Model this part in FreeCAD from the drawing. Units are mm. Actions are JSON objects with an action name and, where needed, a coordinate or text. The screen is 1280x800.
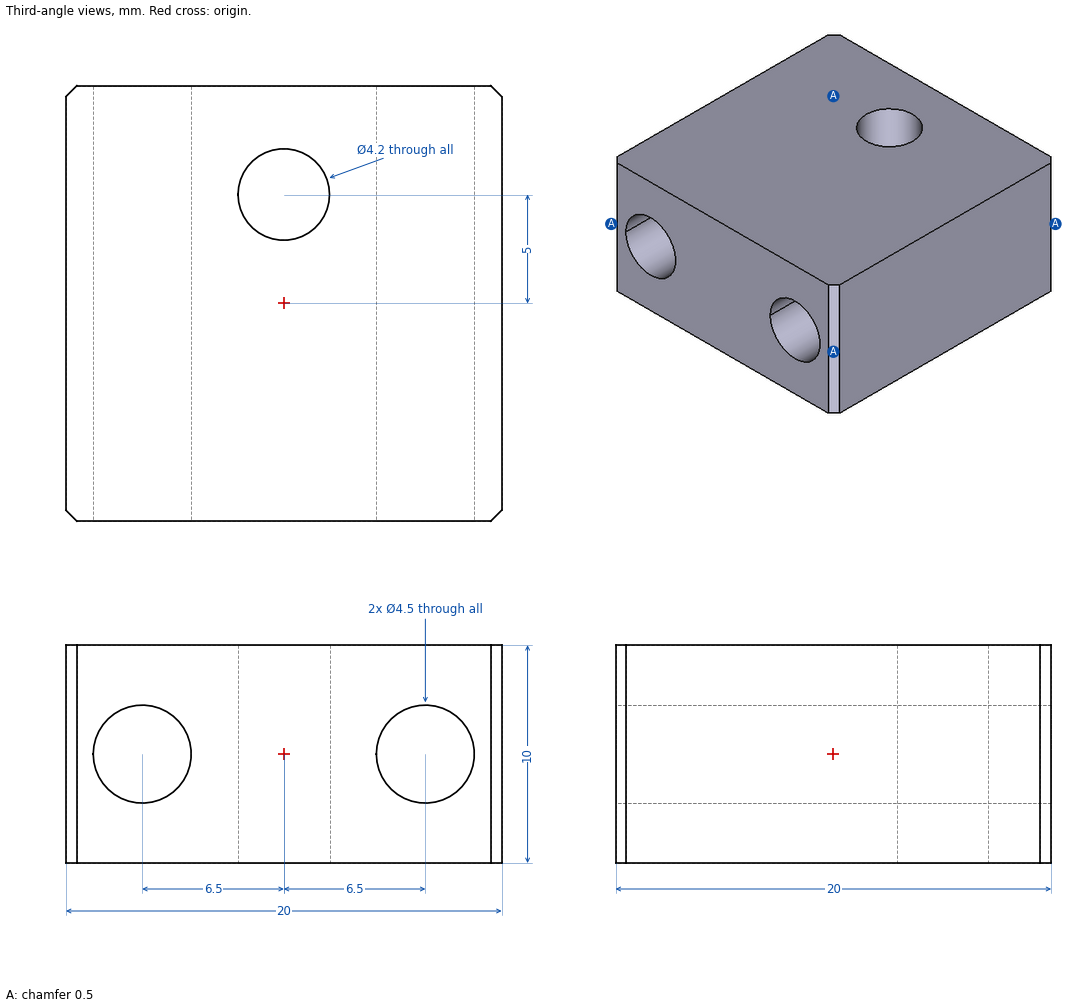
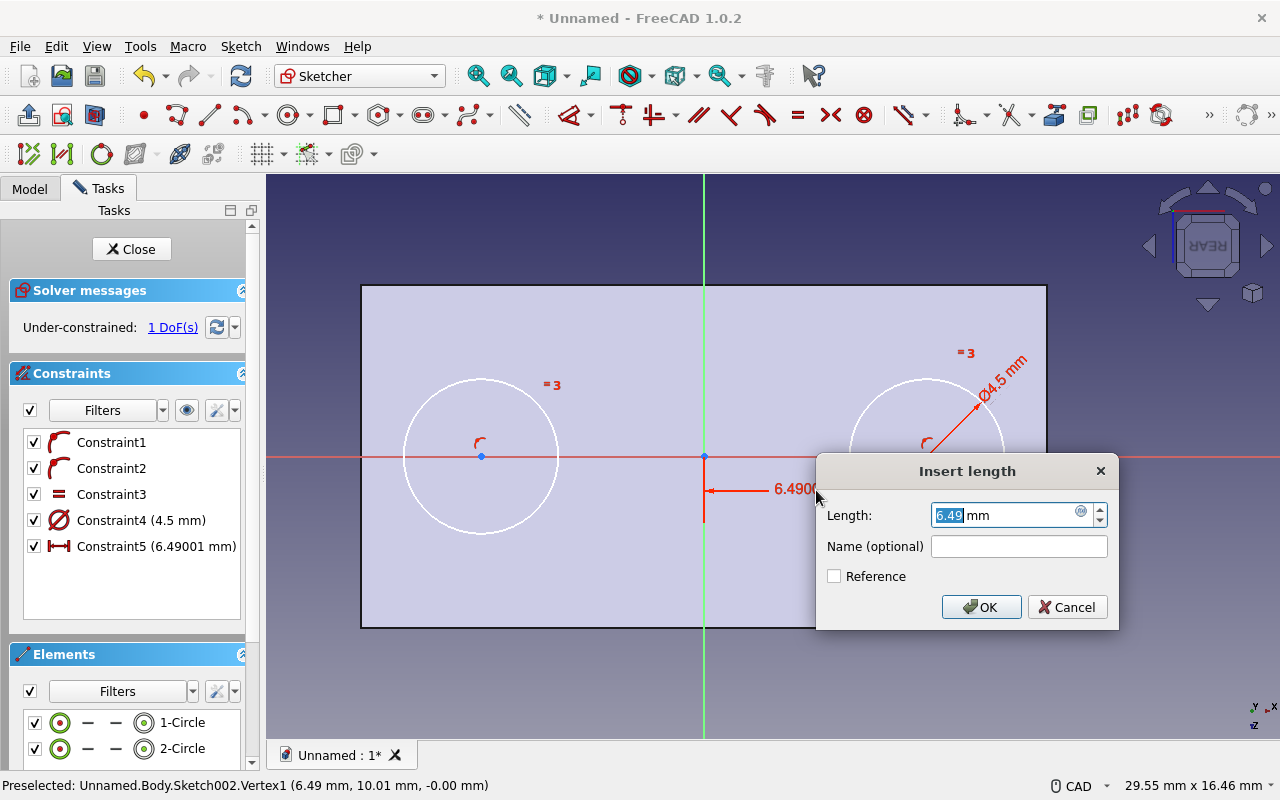
{"action": "type", "text": "6.5"}
{"action": "key", "text": "Return"}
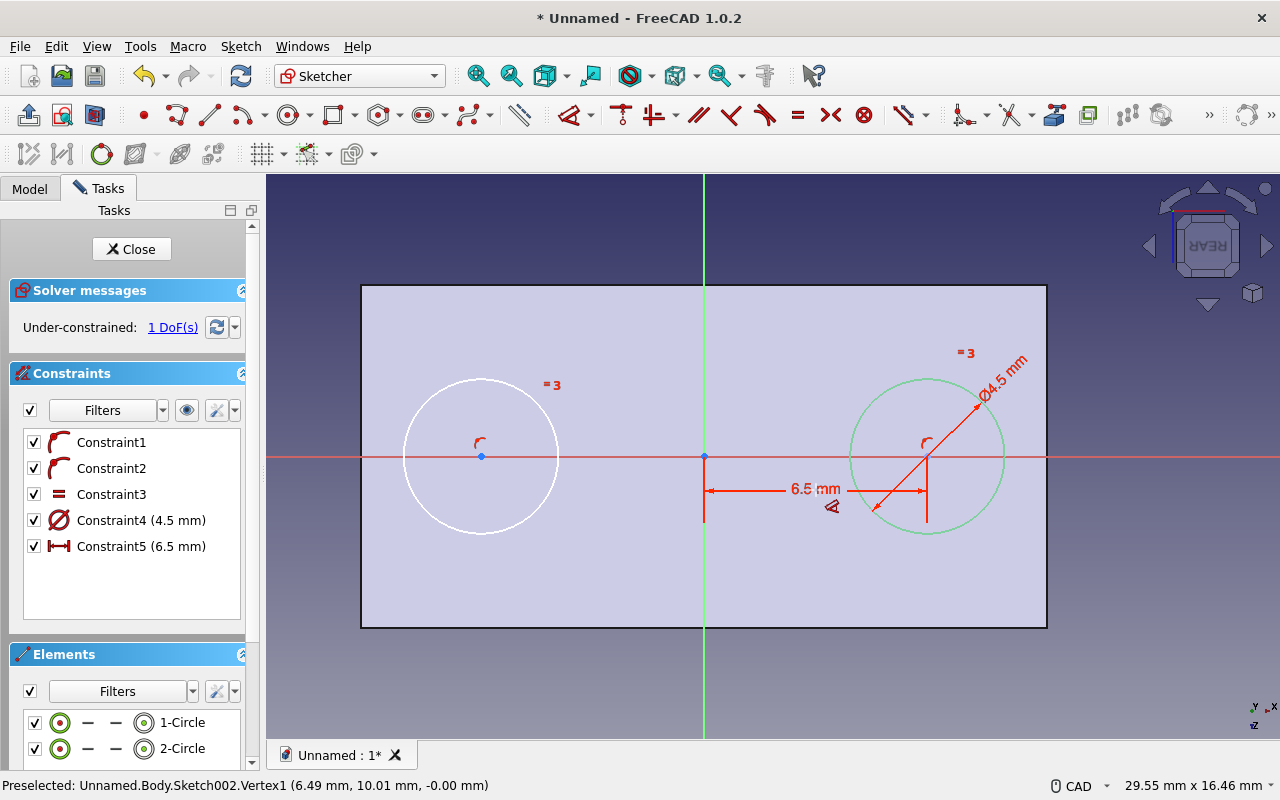
{"action": "left_click", "coordinate": [481, 456]}
{"action": "left_click", "coordinate": [593, 490]}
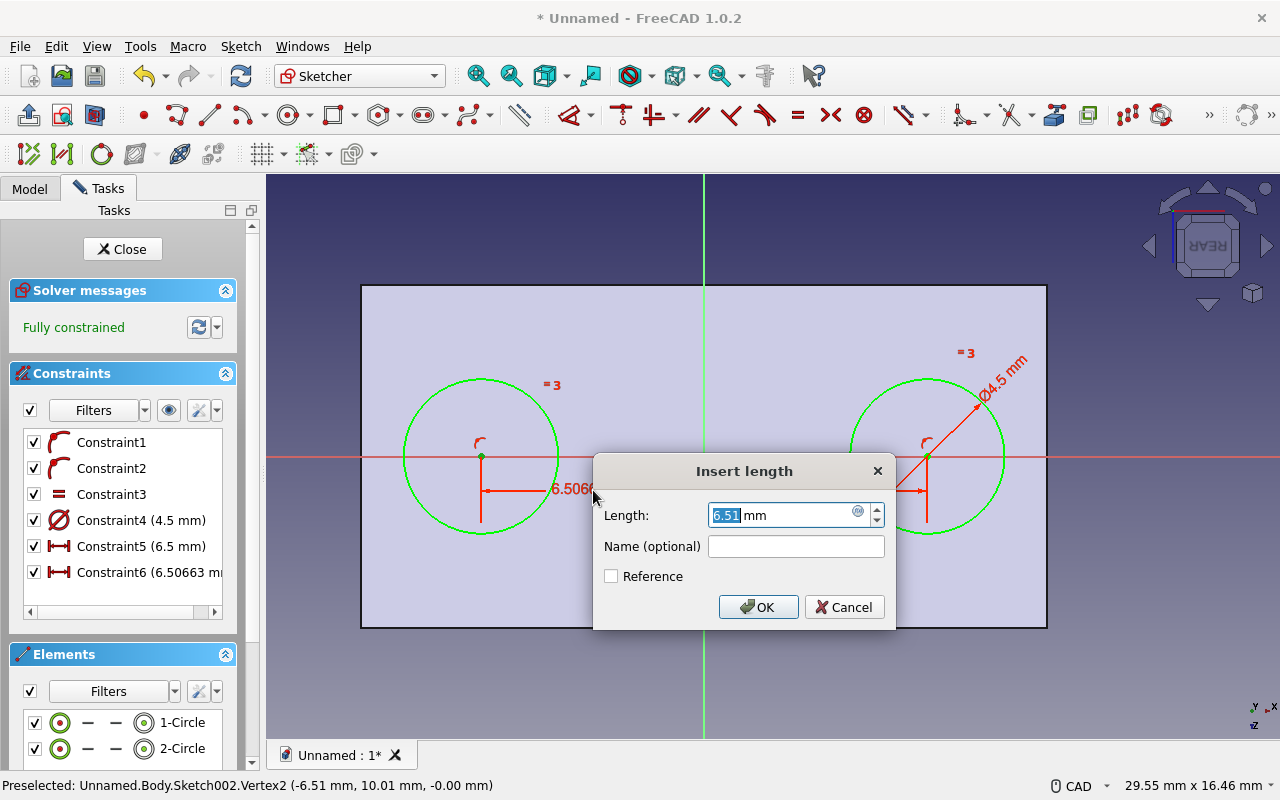
{"action": "type", "text": "6.5"}
{"action": "key", "text": "Return"}
{"action": "key", "text": "Escape"}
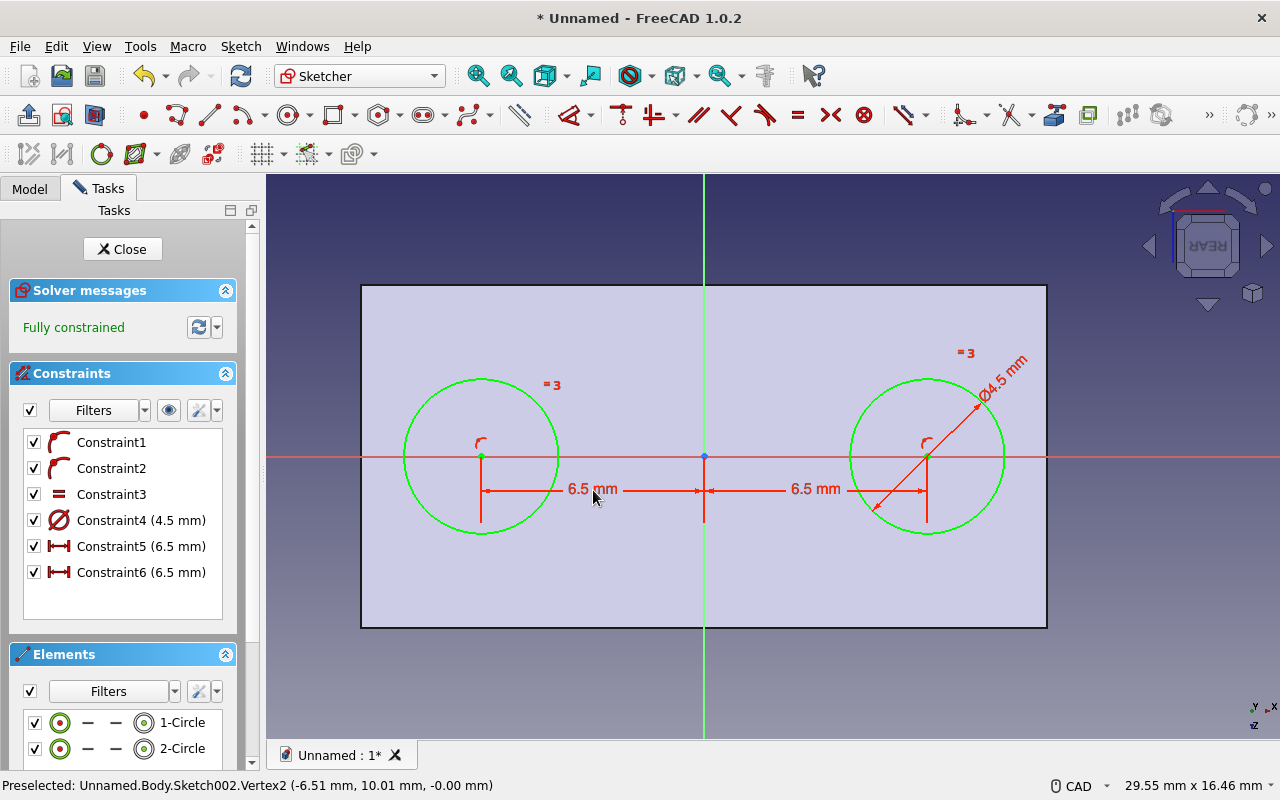
{"action": "left_click", "coordinate": [123, 249]}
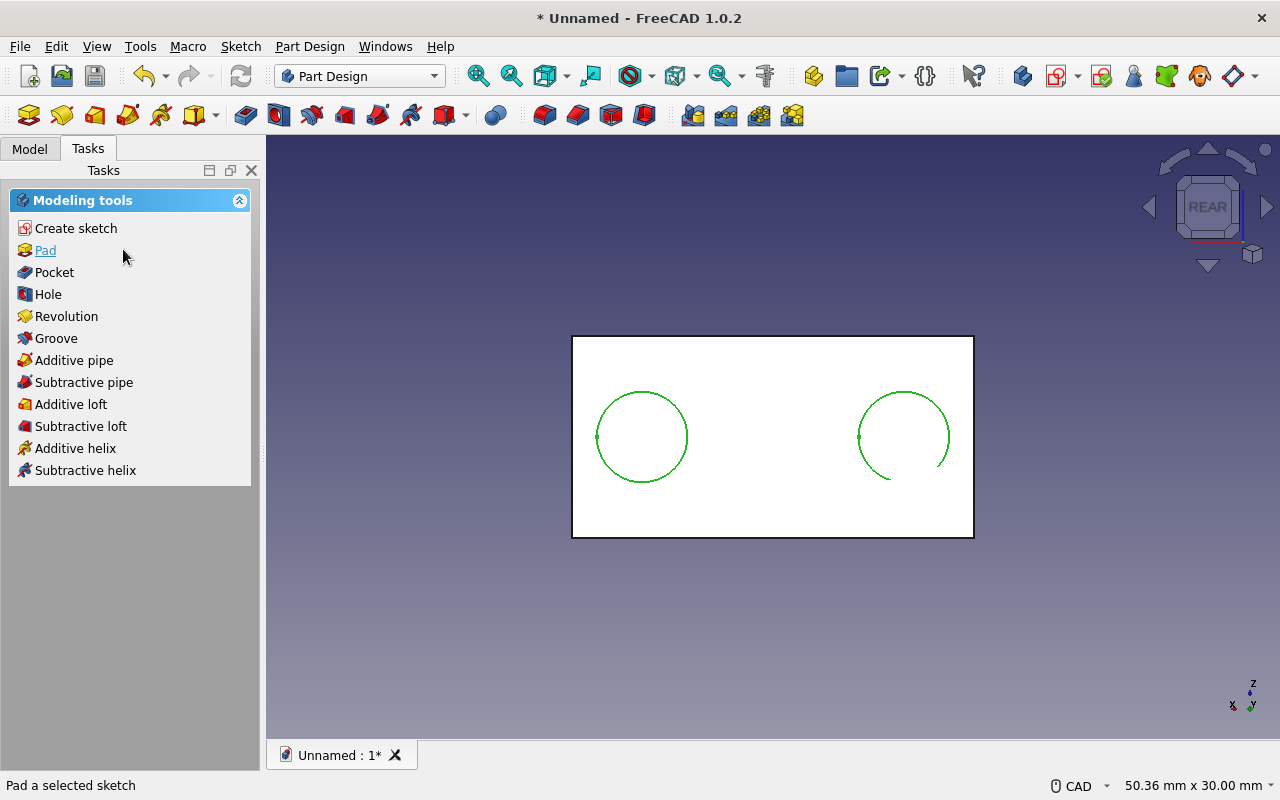
{"action": "left_click", "coordinate": [279, 116]}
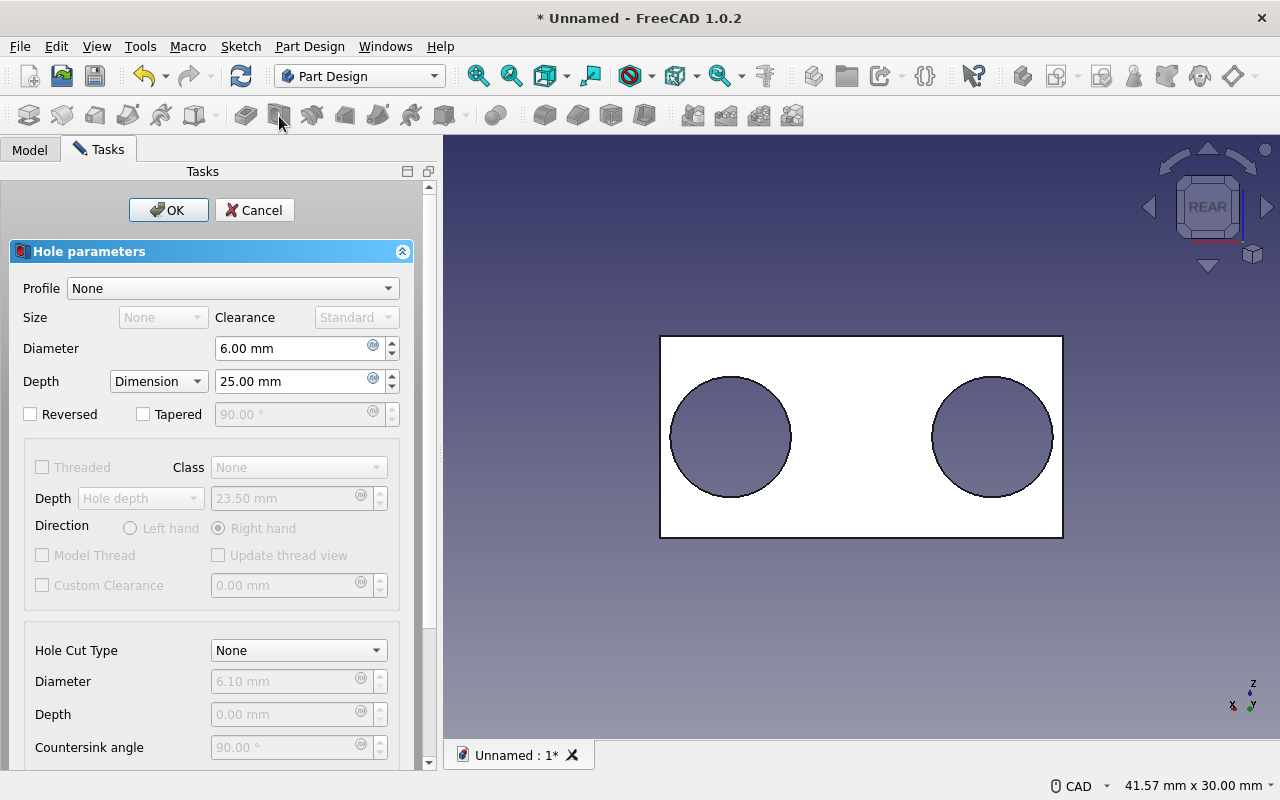
{"action": "triple_click", "coordinate": [300, 348]}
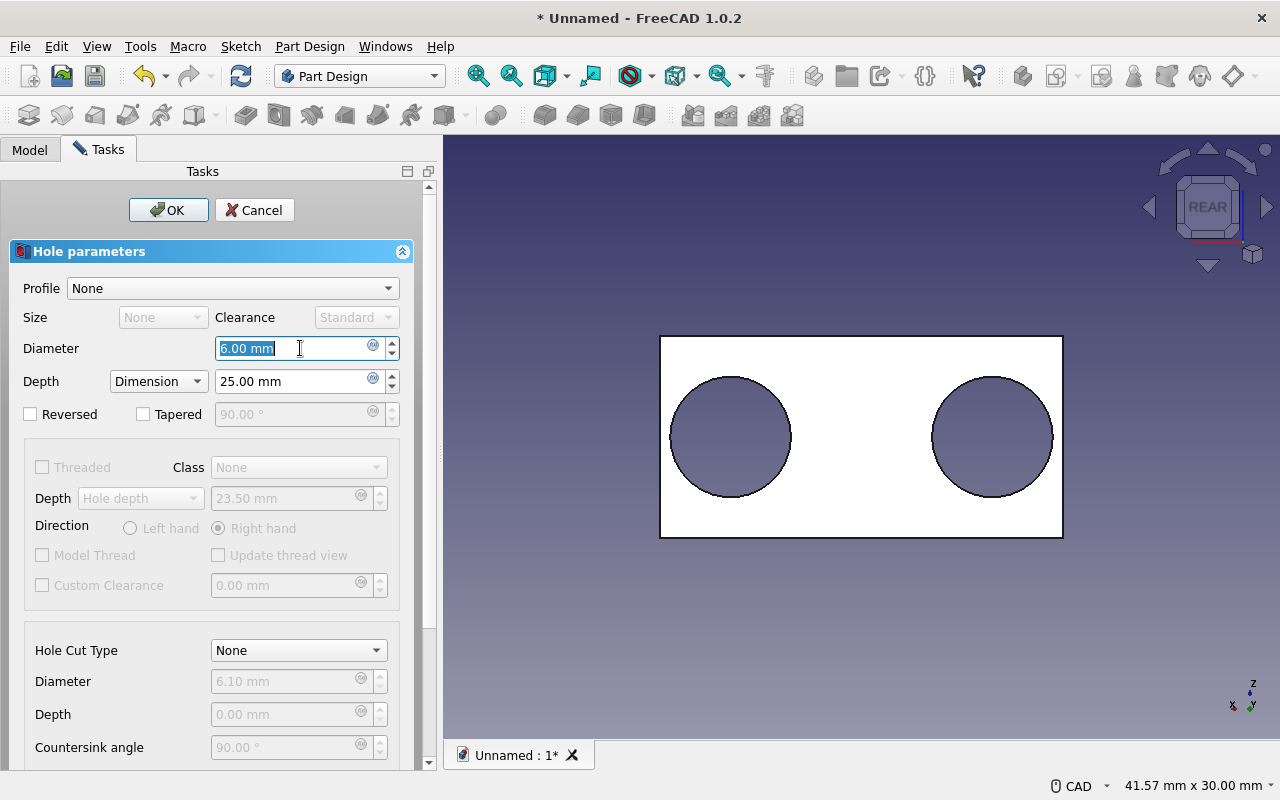
{"action": "type", "text": "4.5"}
{"action": "key", "text": "Tab"}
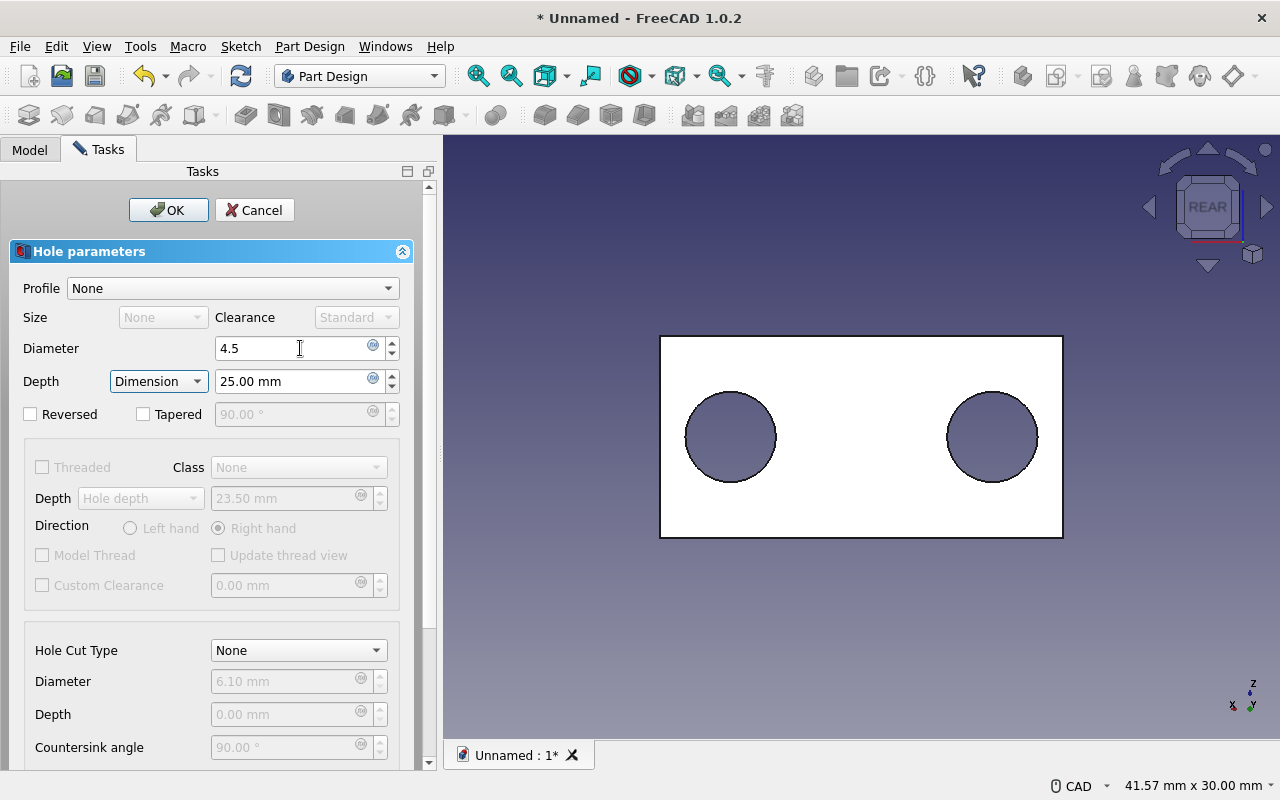
{"action": "left_click", "coordinate": [160, 382]}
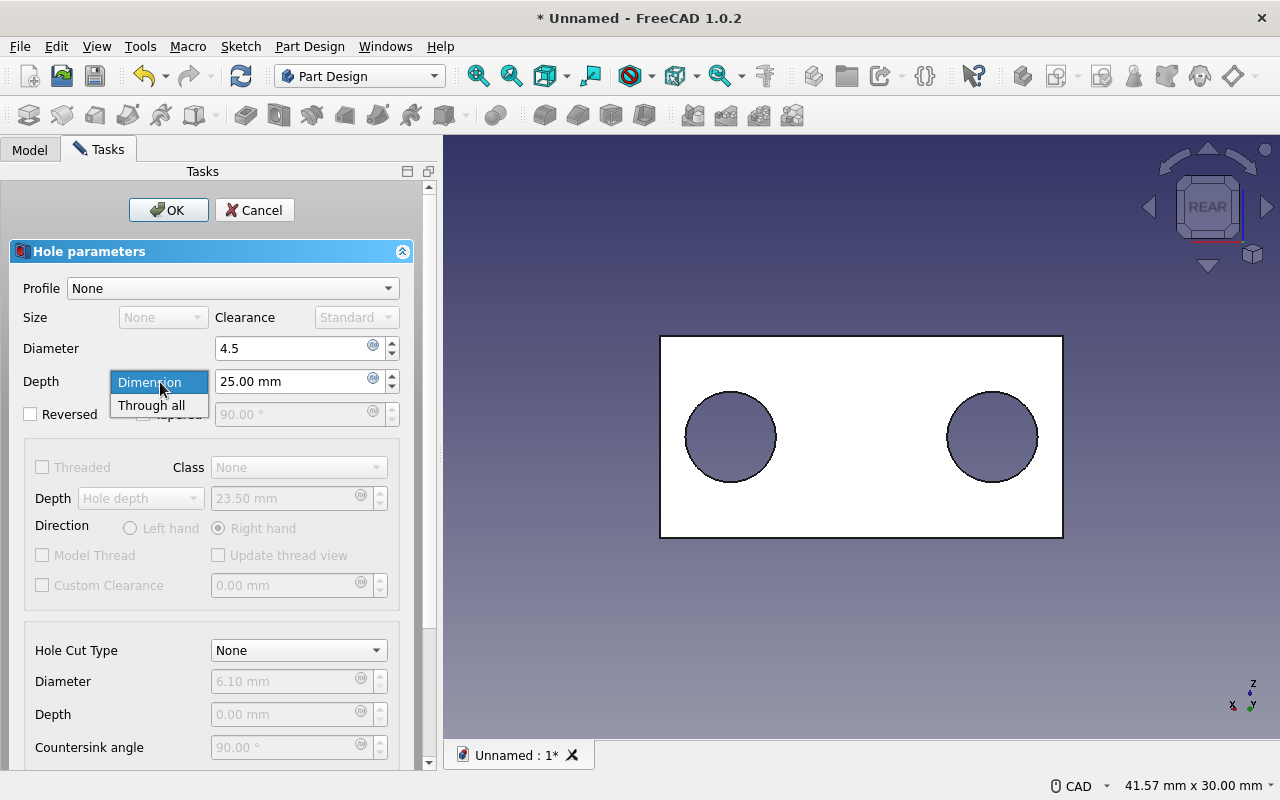
{"action": "left_click", "coordinate": [158, 406]}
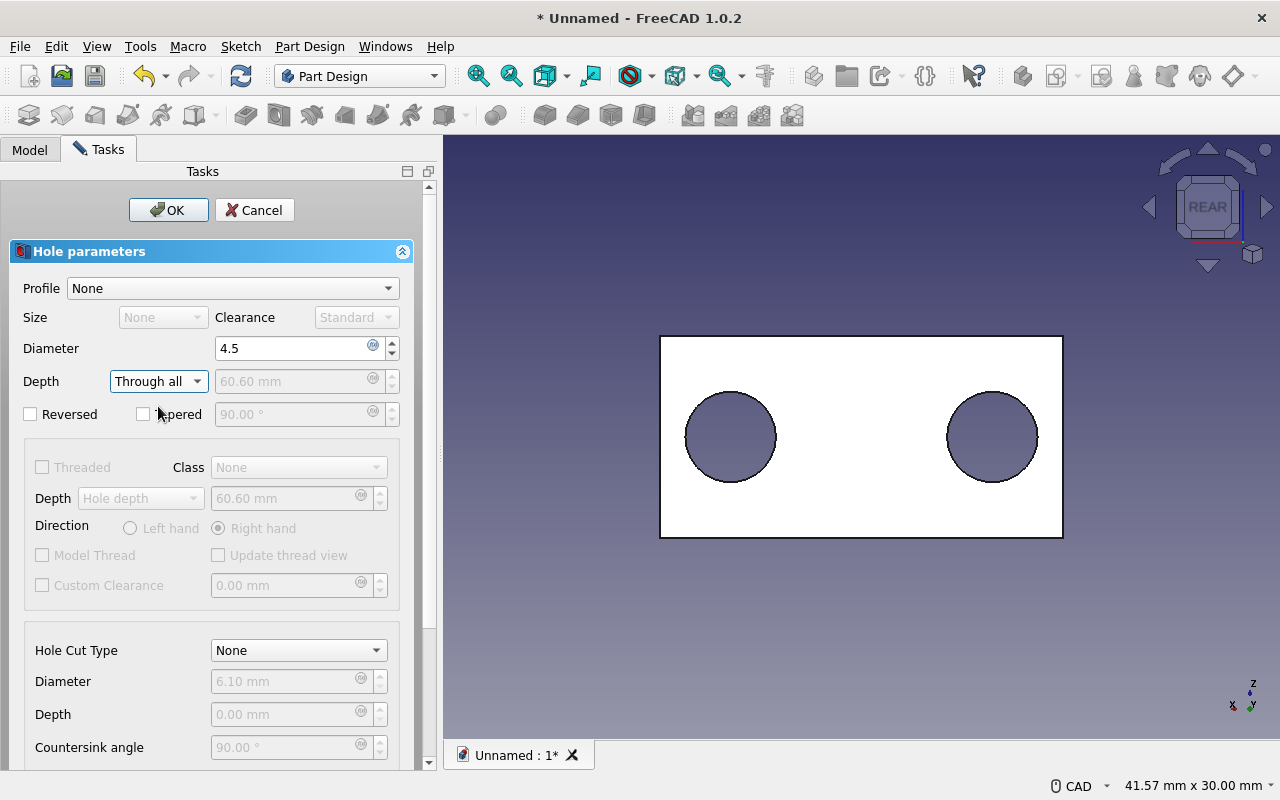
{"action": "left_click", "coordinate": [169, 210]}